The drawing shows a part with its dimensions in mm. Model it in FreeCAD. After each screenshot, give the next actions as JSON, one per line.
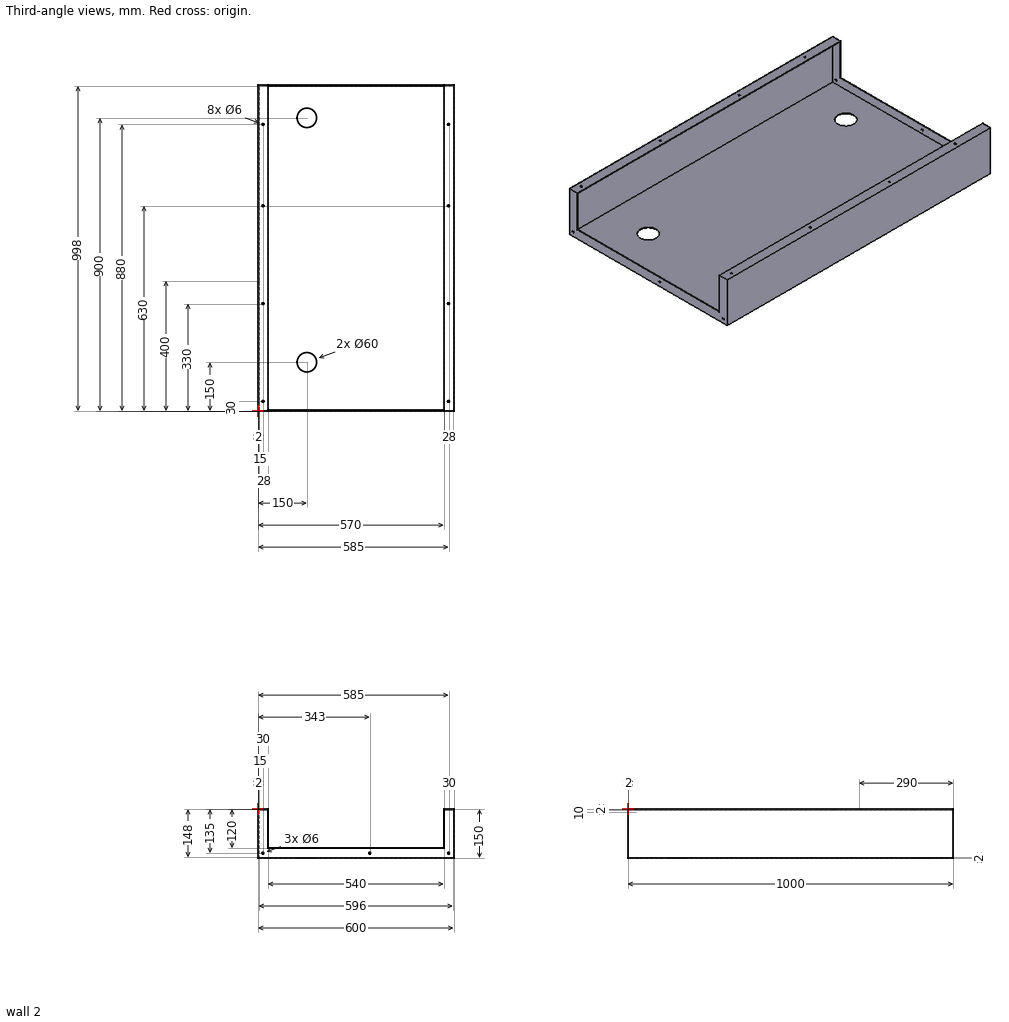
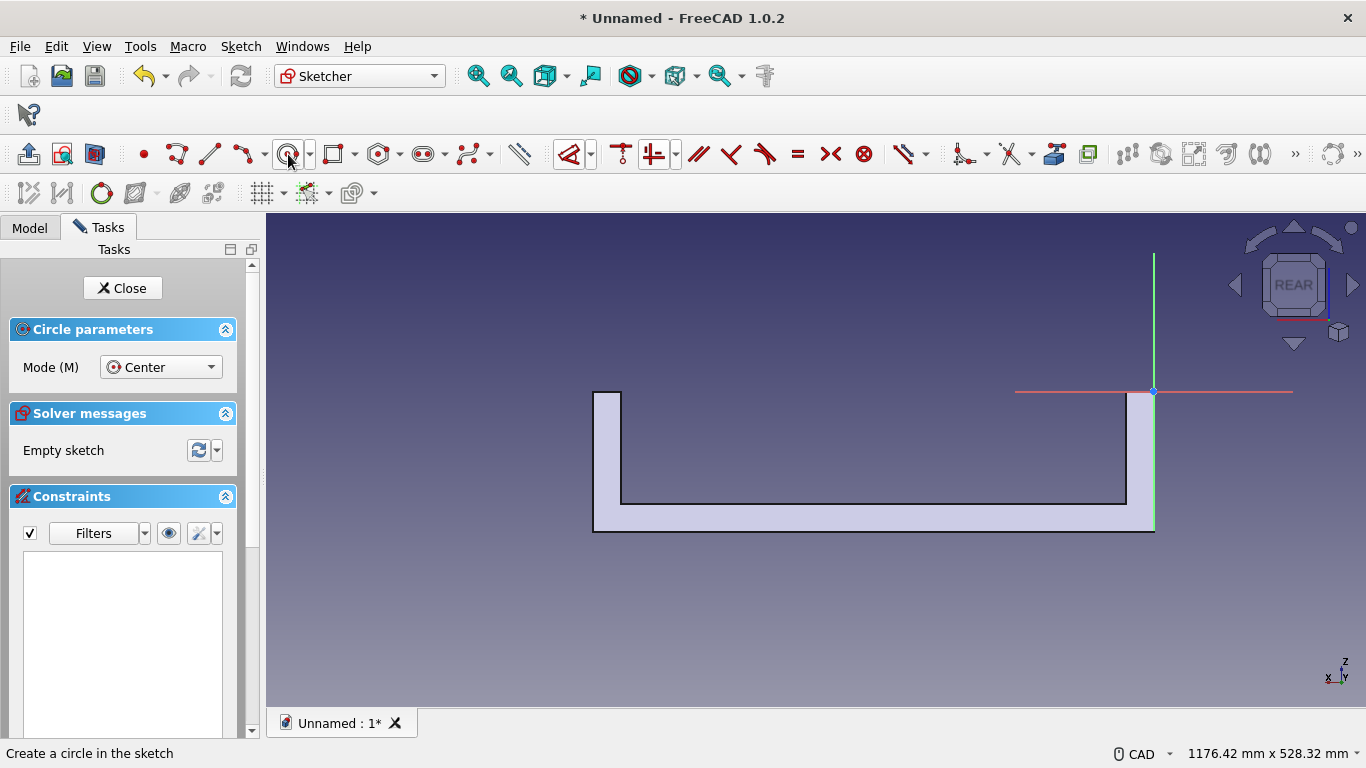
{"action": "scroll", "coordinate": [1140, 518], "scroll_direction": "up", "scroll_amount": 11}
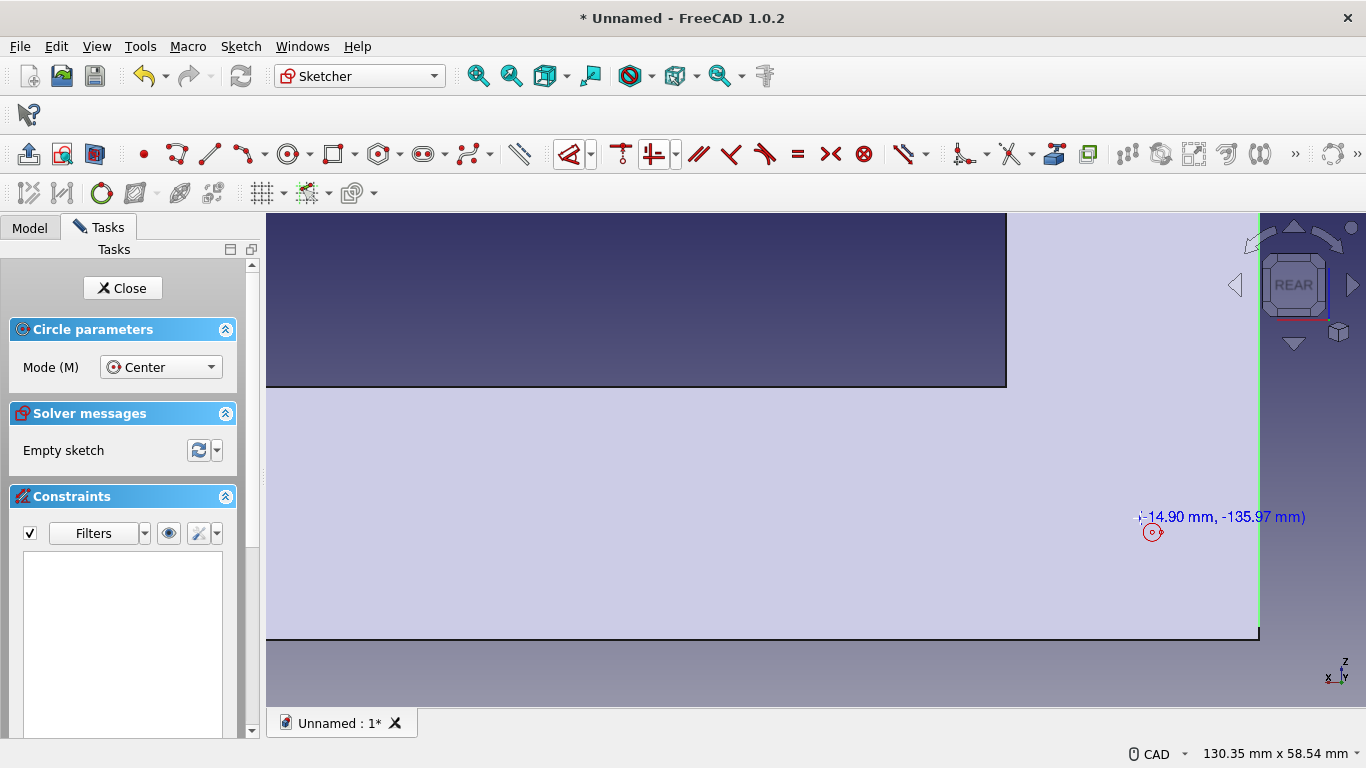
{"action": "scroll", "coordinate": [1056, 539], "scroll_direction": "down", "scroll_amount": 10}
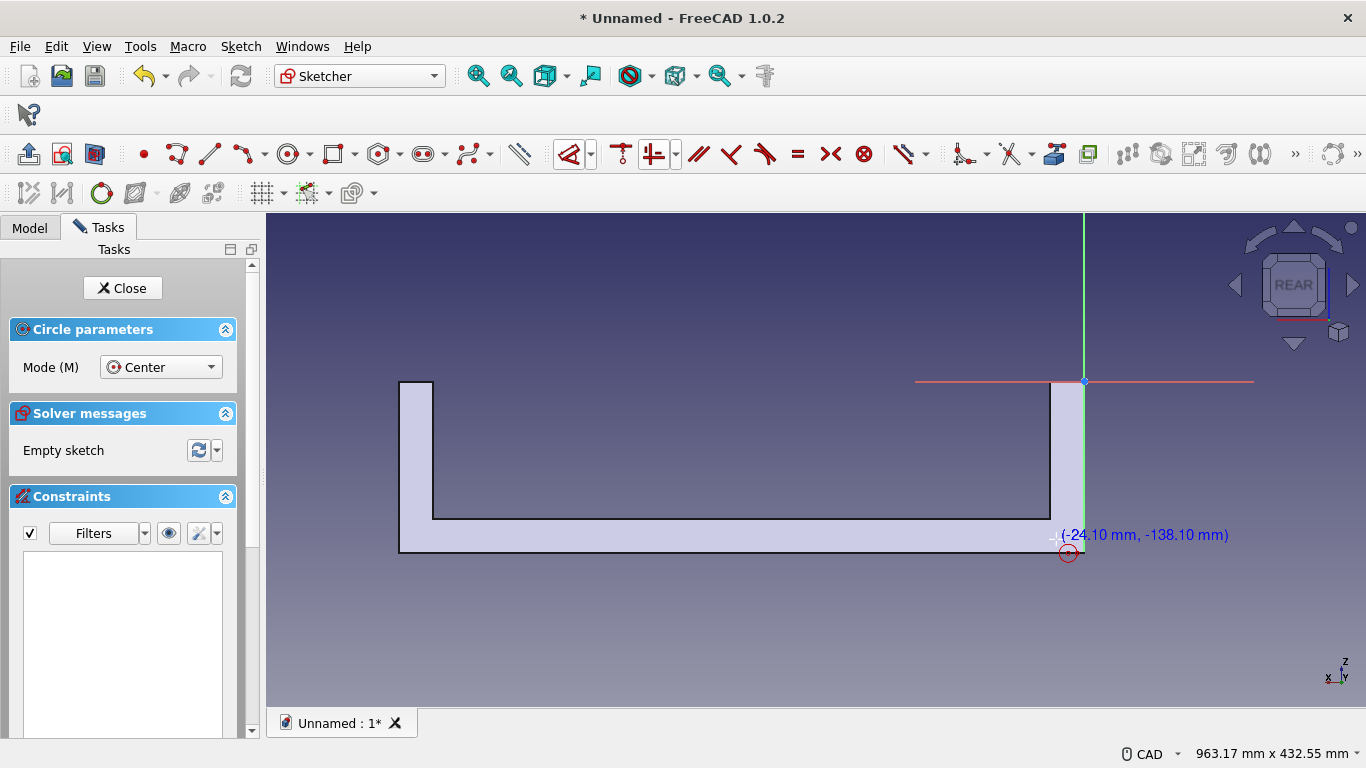
{"action": "left_click", "coordinate": [1067, 536]}
{"action": "mouse_move", "coordinate": [1069, 534]}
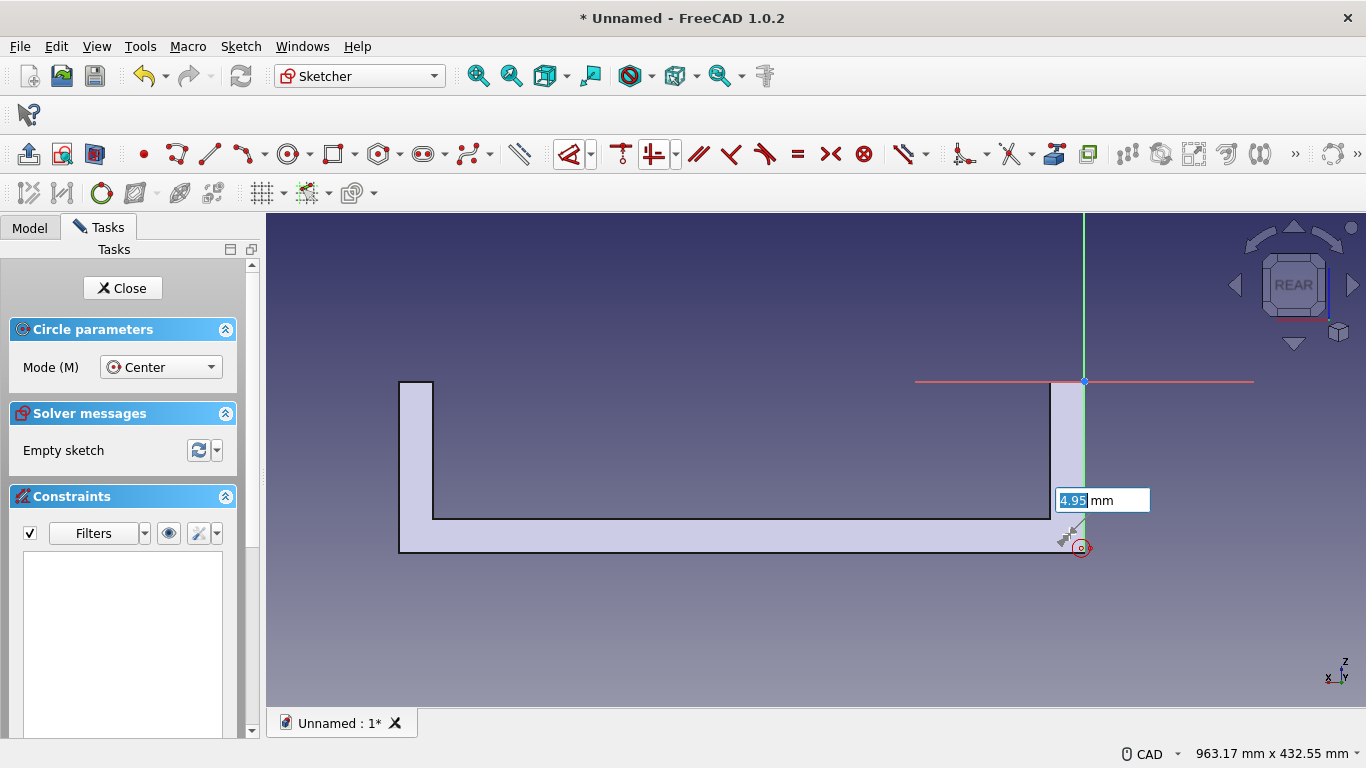
{"action": "type", "text": "6"}
{"action": "key", "text": "Return"}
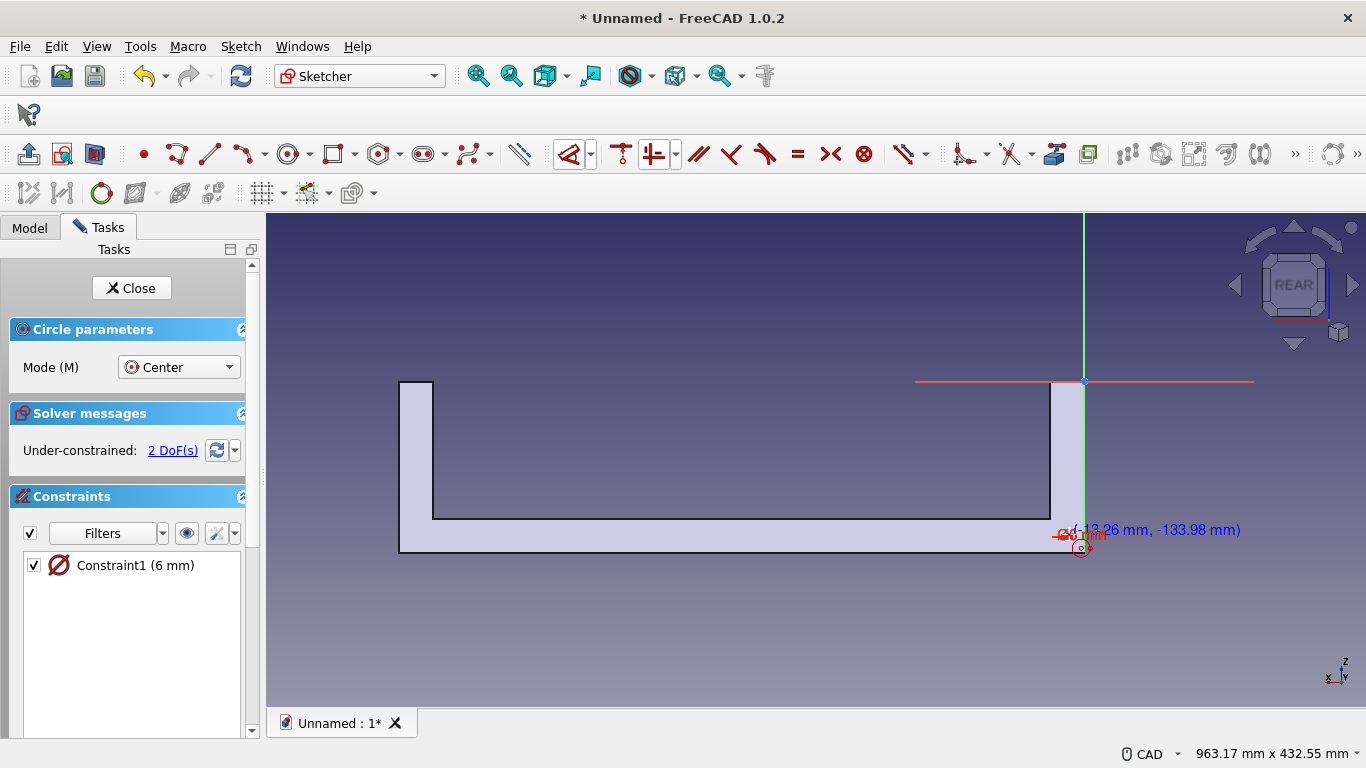
{"action": "scroll", "coordinate": [692, 536], "scroll_direction": "up", "scroll_amount": 10}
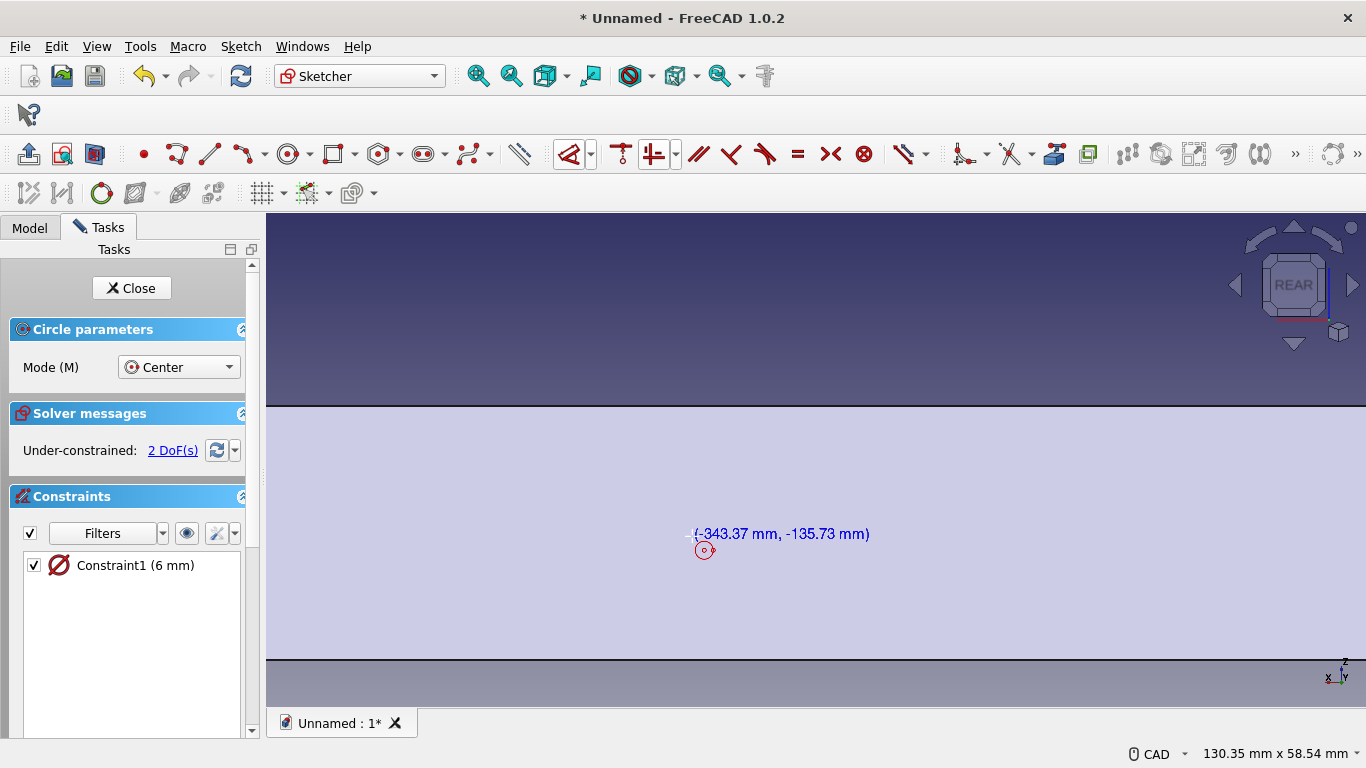
{"action": "scroll", "coordinate": [691, 536], "scroll_direction": "down", "scroll_amount": 10}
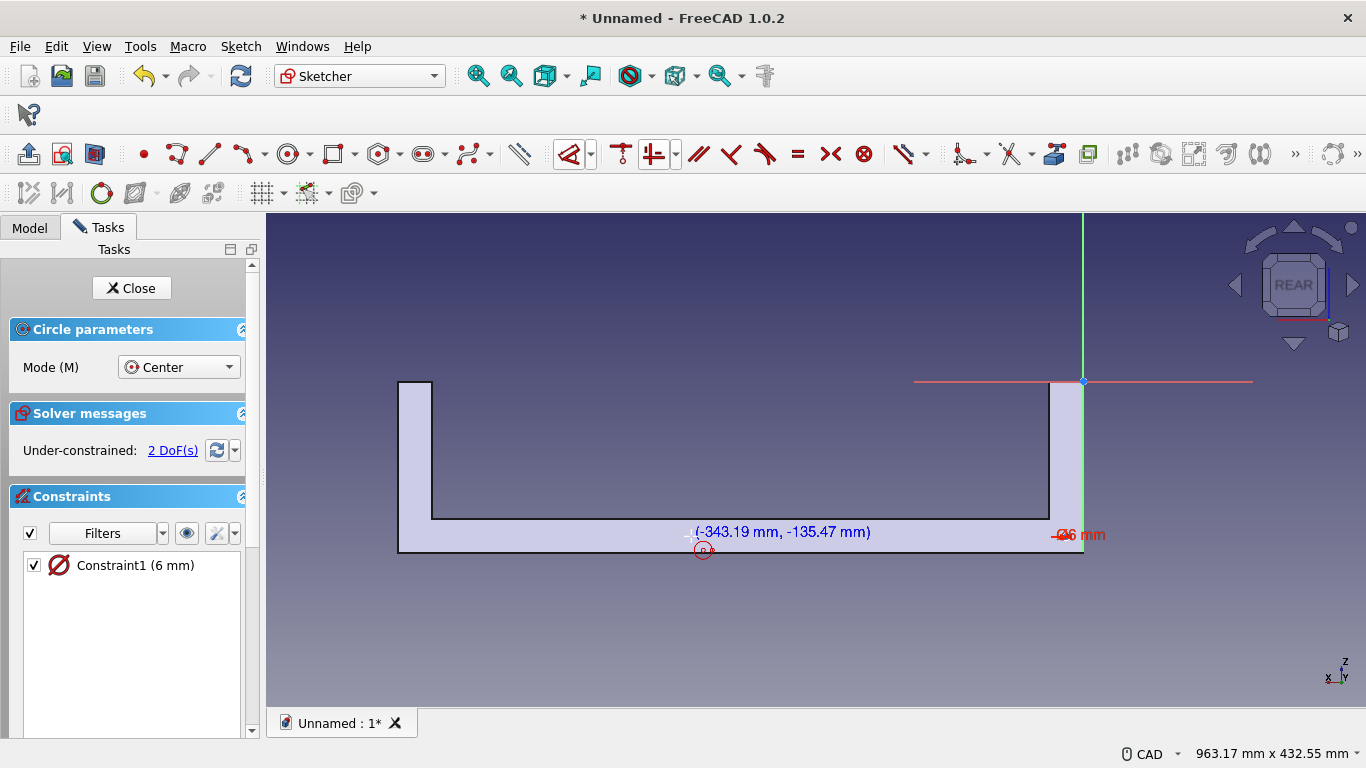
{"action": "left_click", "coordinate": [692, 536]}
{"action": "mouse_move", "coordinate": [694, 534]}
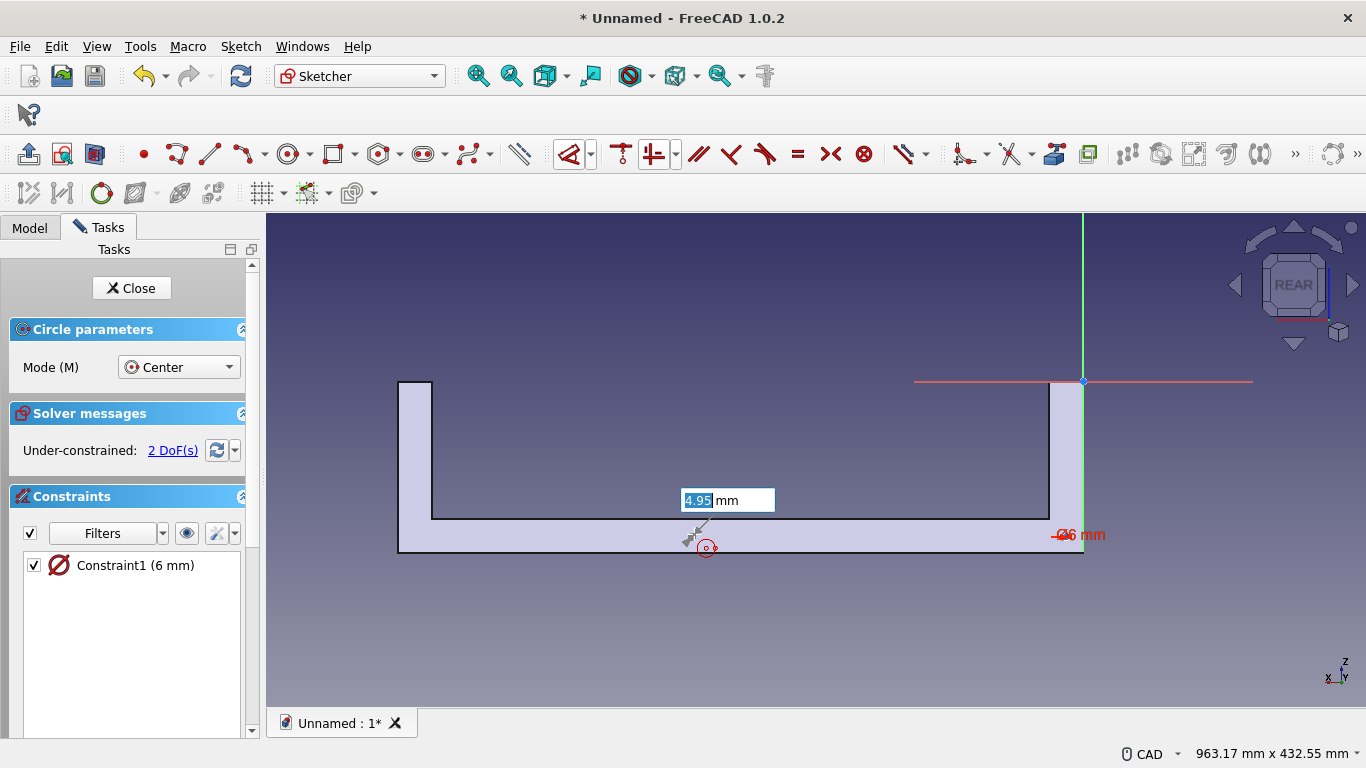
{"action": "type", "text": "6"}
{"action": "key", "text": "Return"}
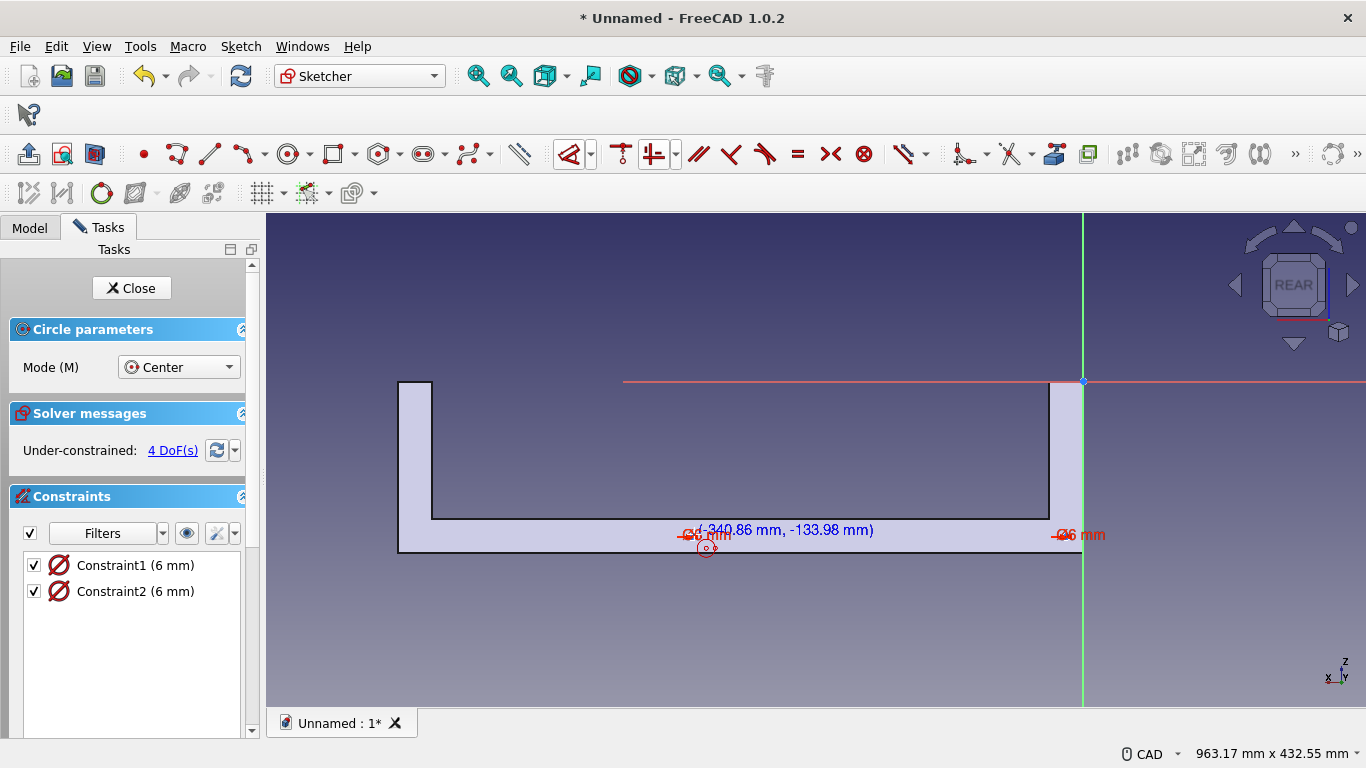
{"action": "scroll", "coordinate": [415, 536], "scroll_direction": "up", "scroll_amount": 10}